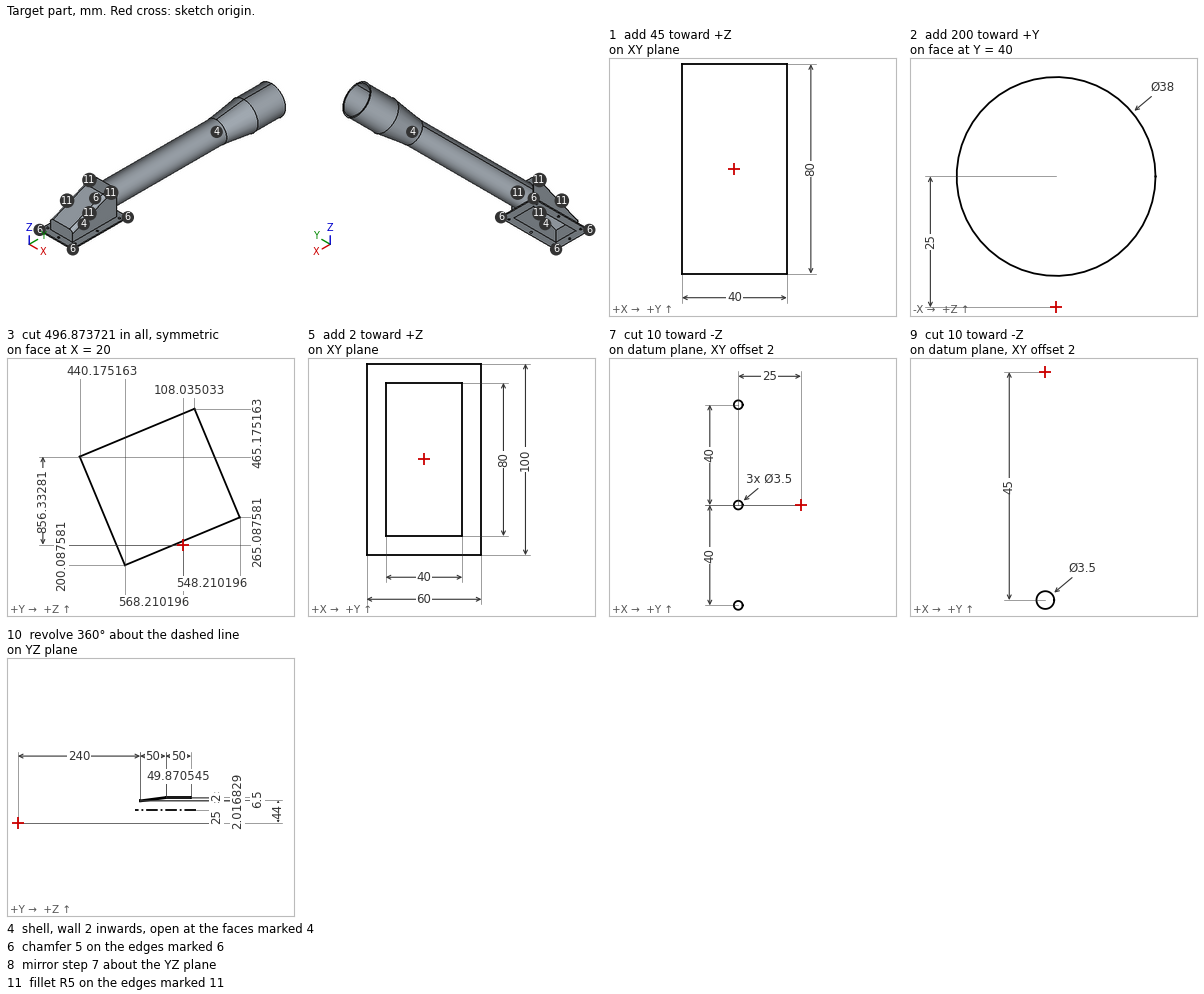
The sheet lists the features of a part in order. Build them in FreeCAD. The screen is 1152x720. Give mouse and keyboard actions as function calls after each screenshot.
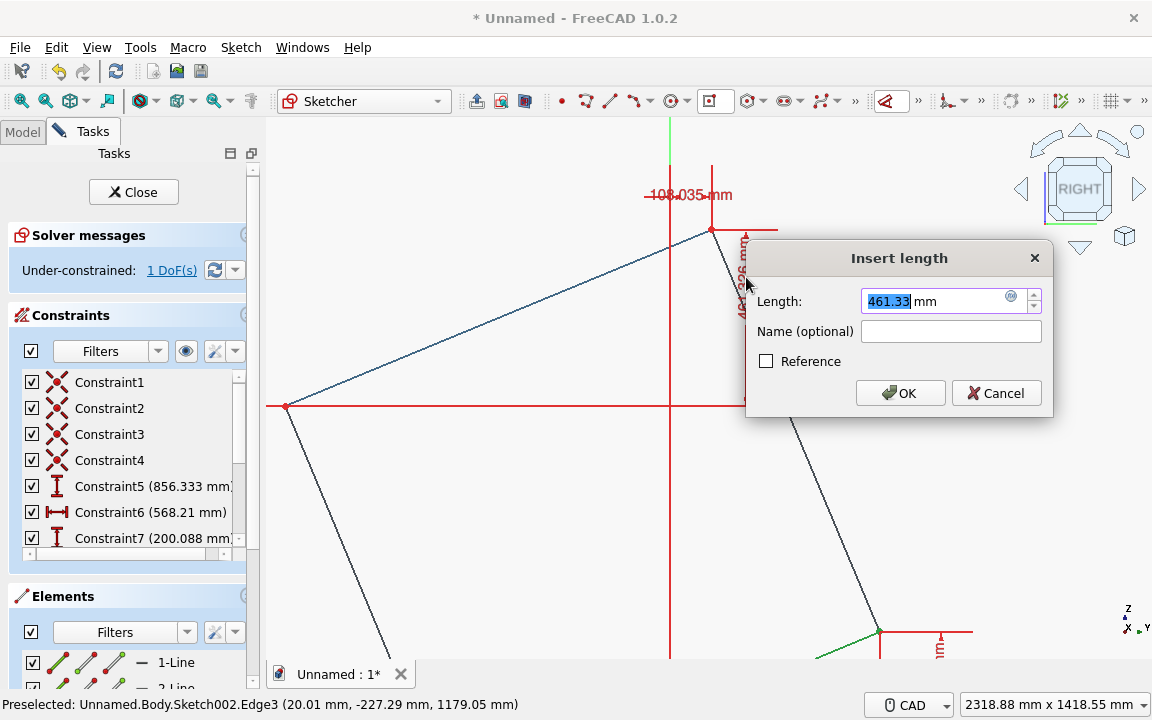
text(465.175163)
key(Return)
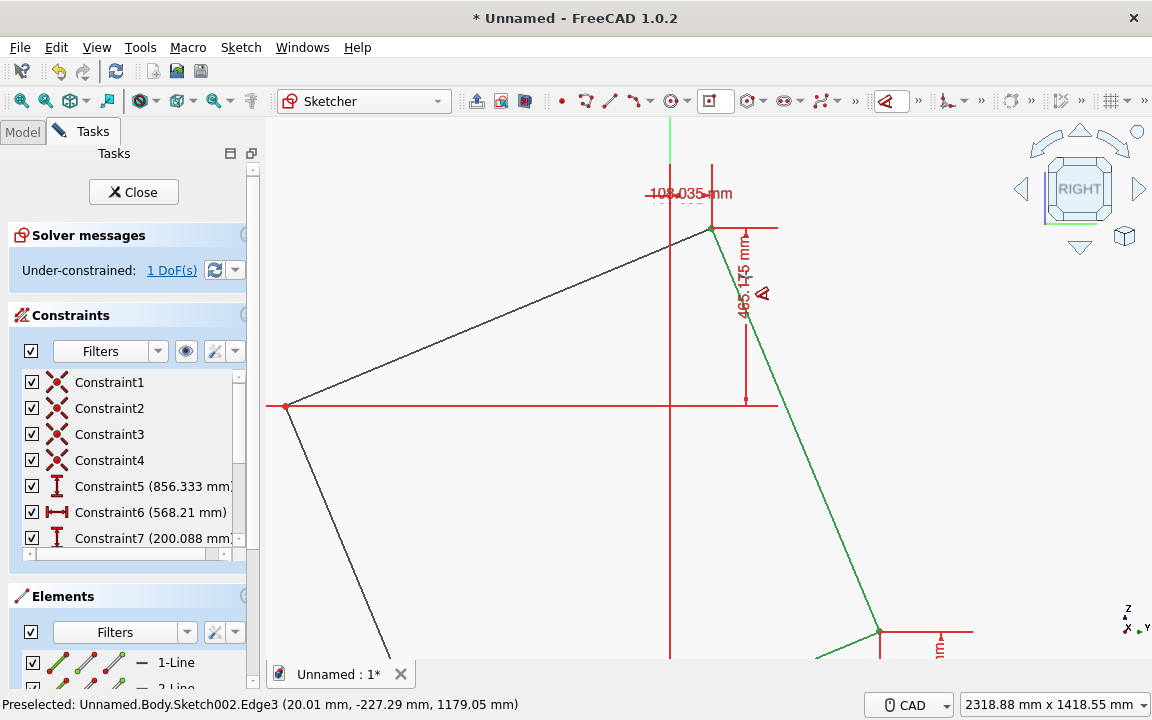
click(336, 527)
click(410, 372)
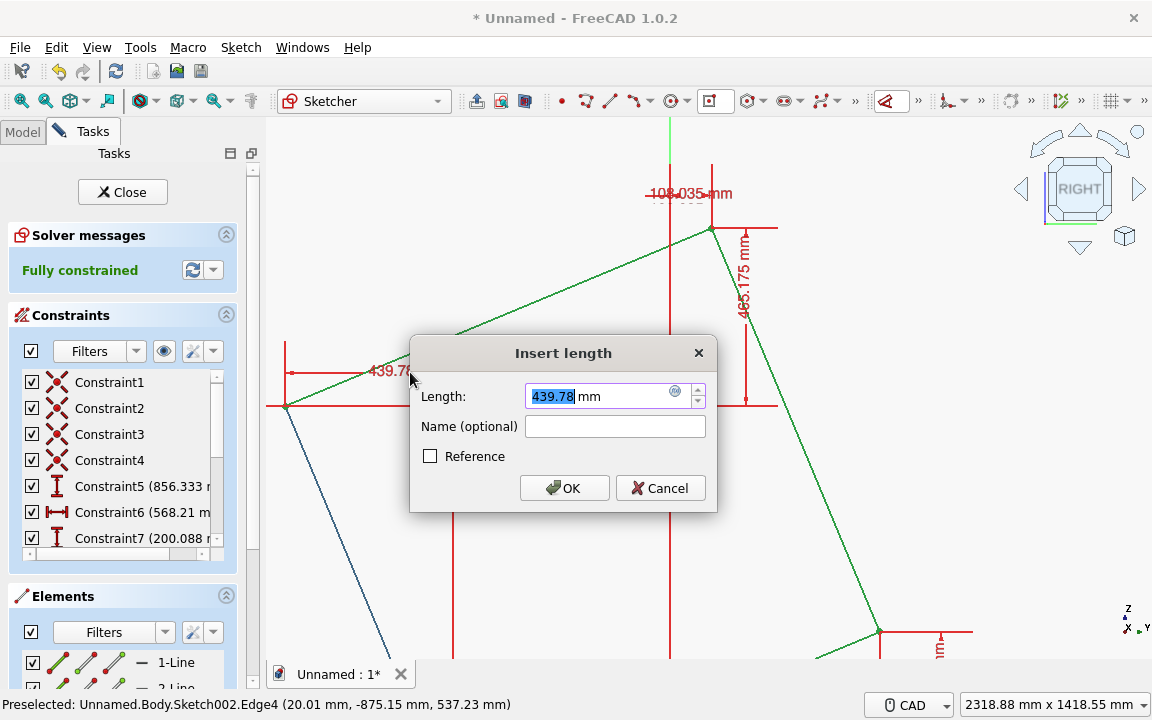
text(440.175163)
key(Return)
key(Escape)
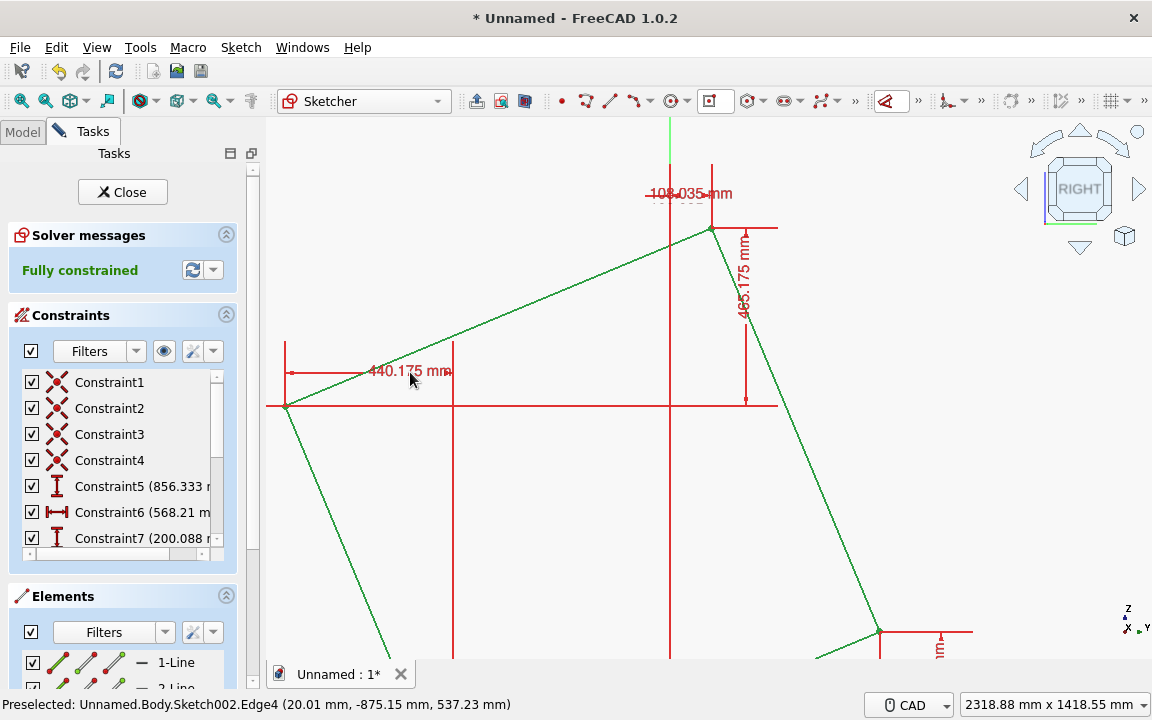
click(123, 192)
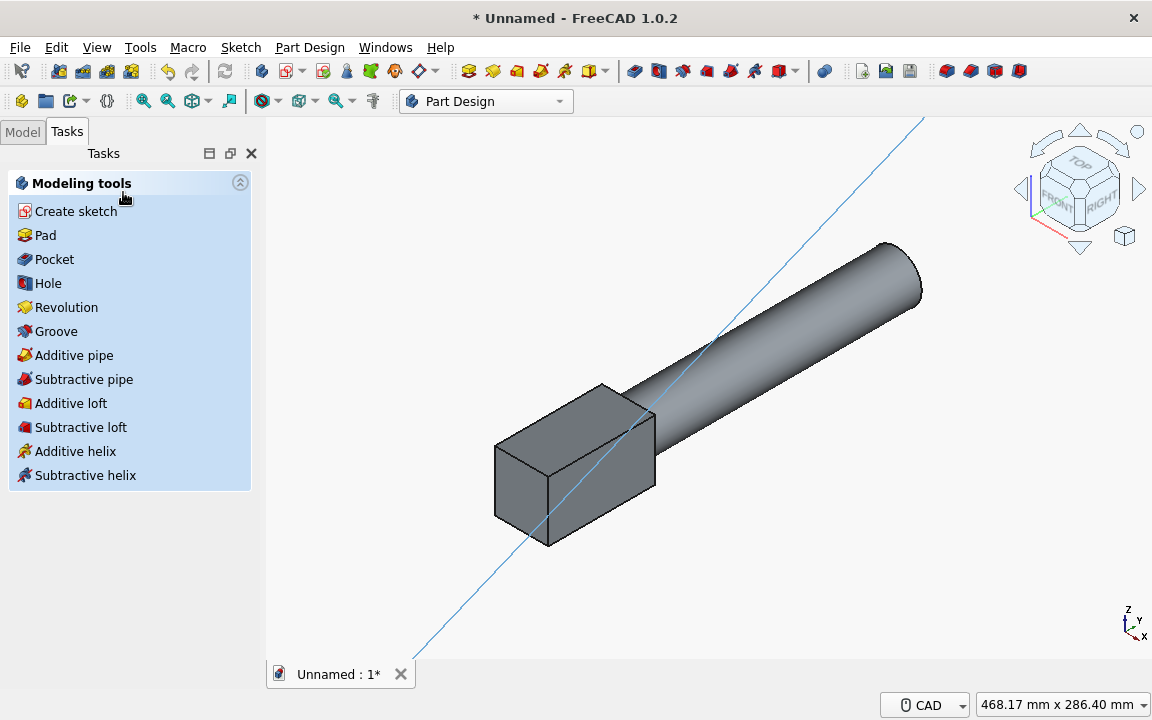
click(636, 72)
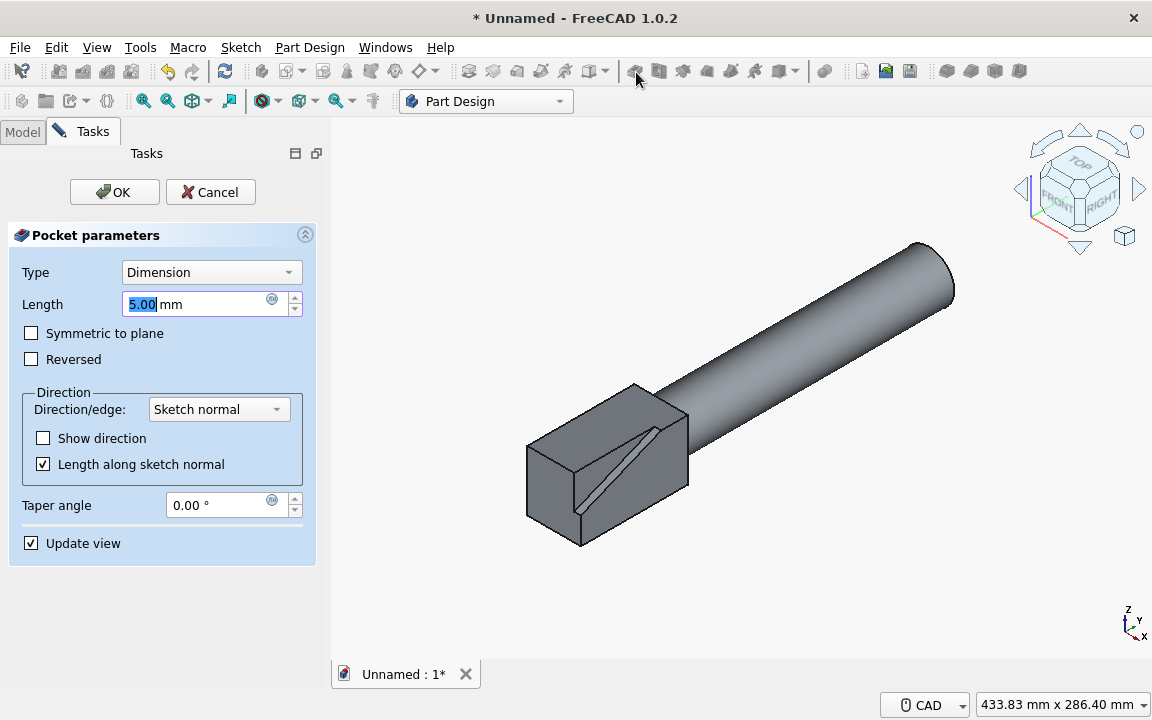
text(496.873721)
key(Tab)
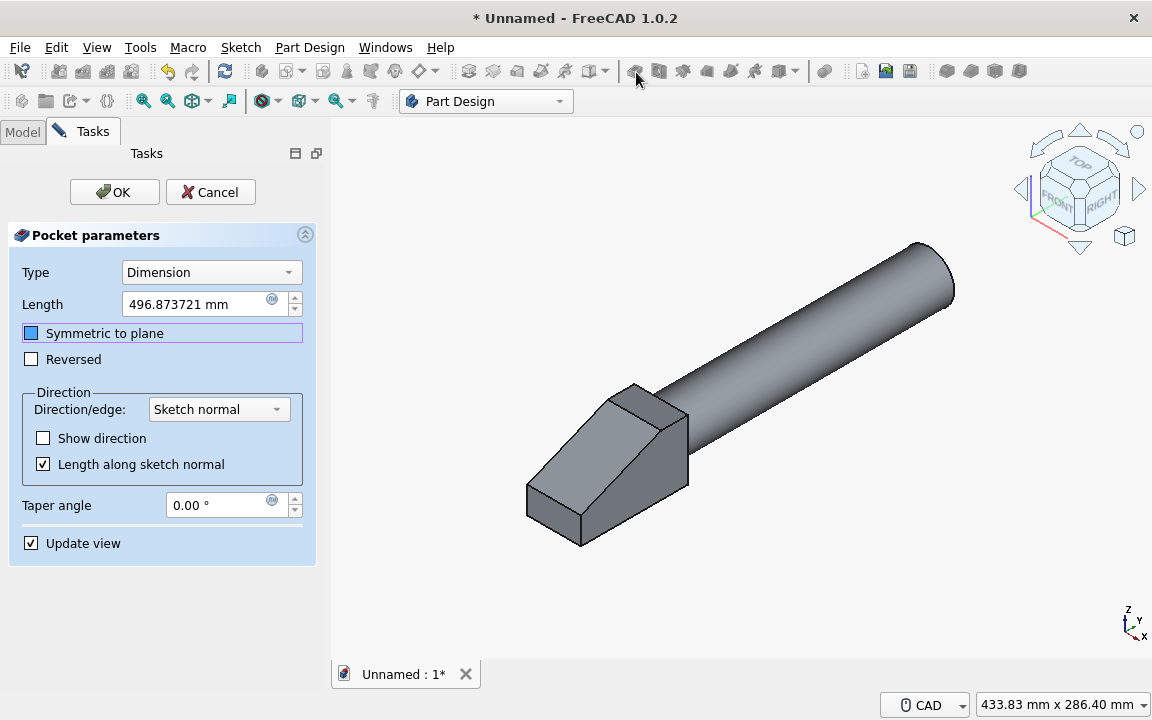
click(30, 333)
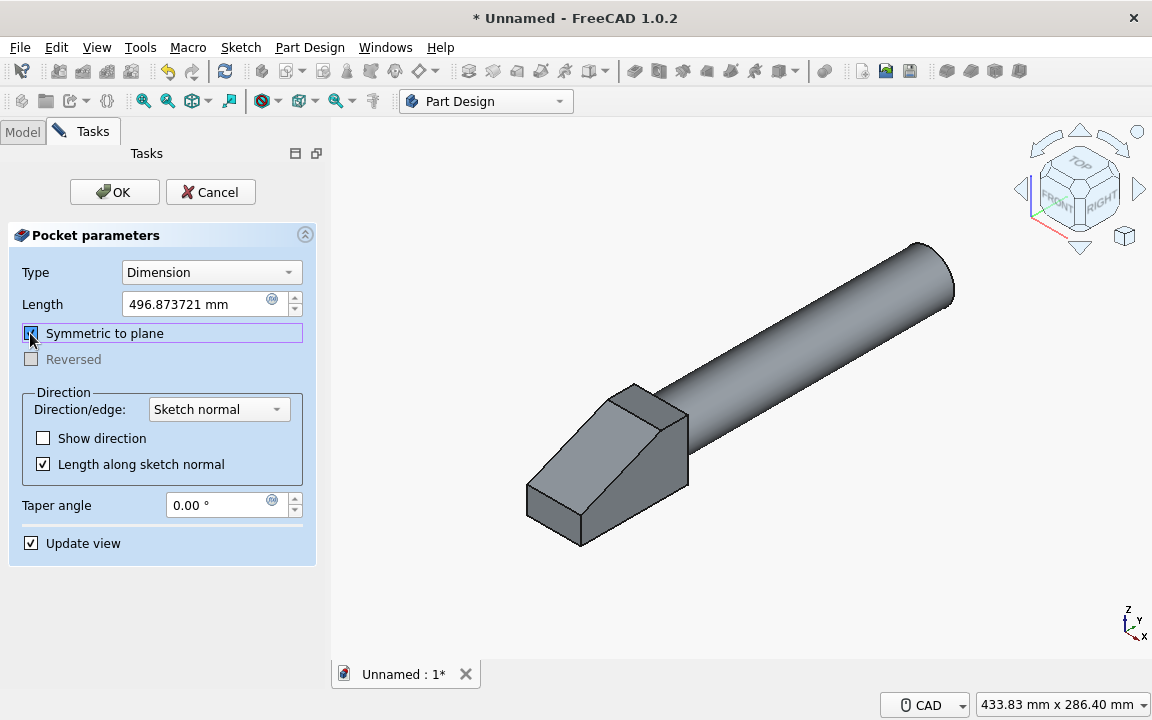
click(115, 192)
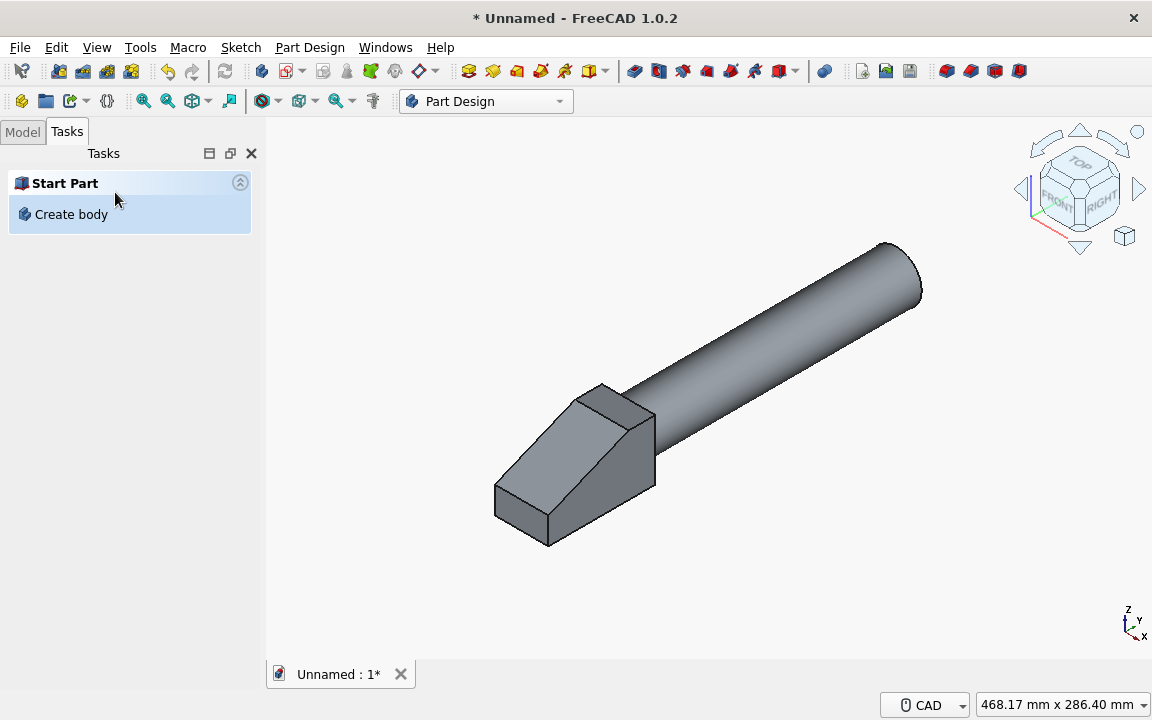
key(2)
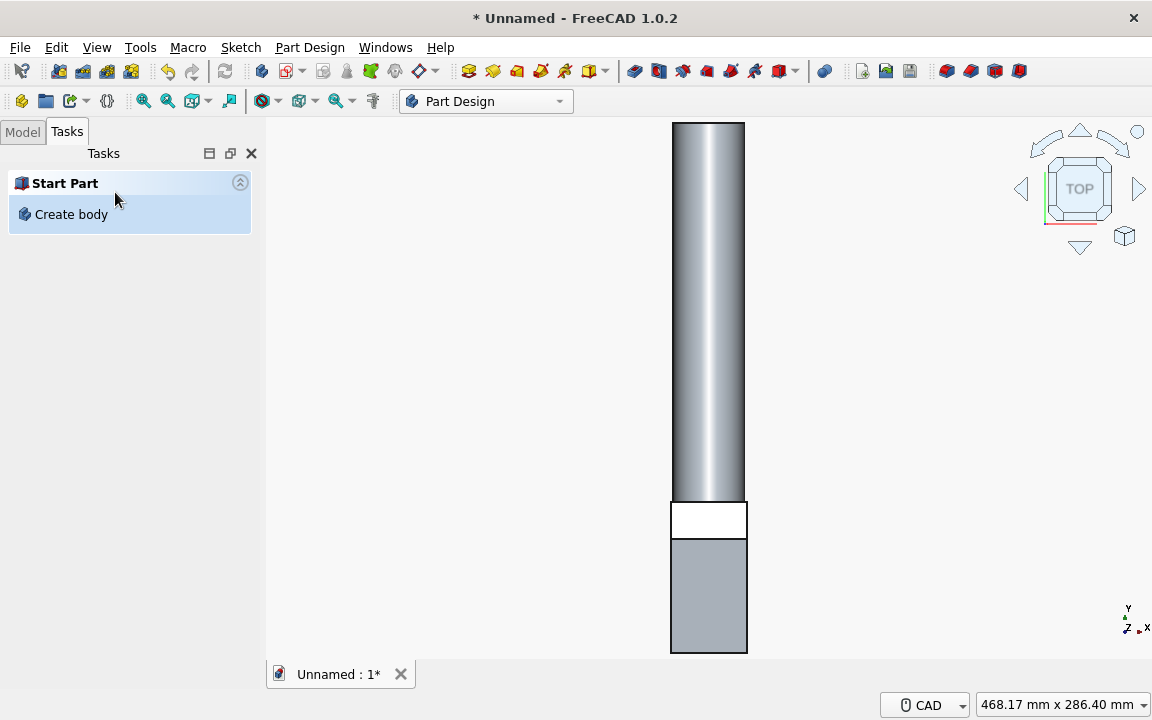
key(0)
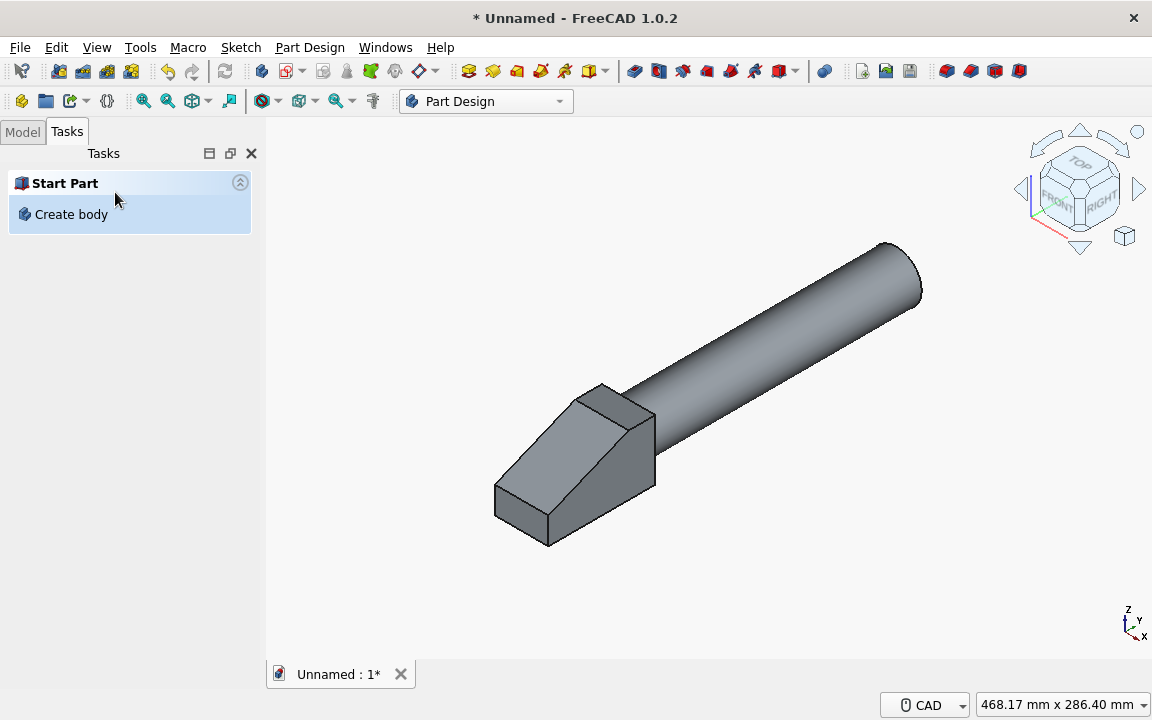
key(1)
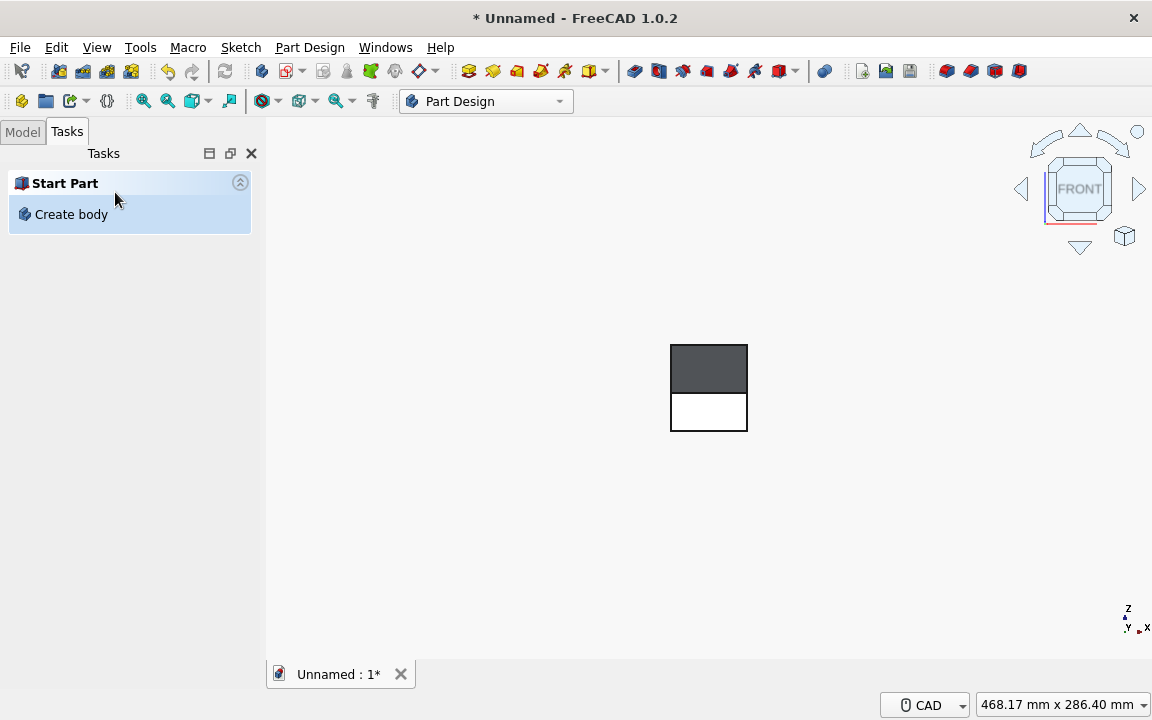
key(v)
key(f)